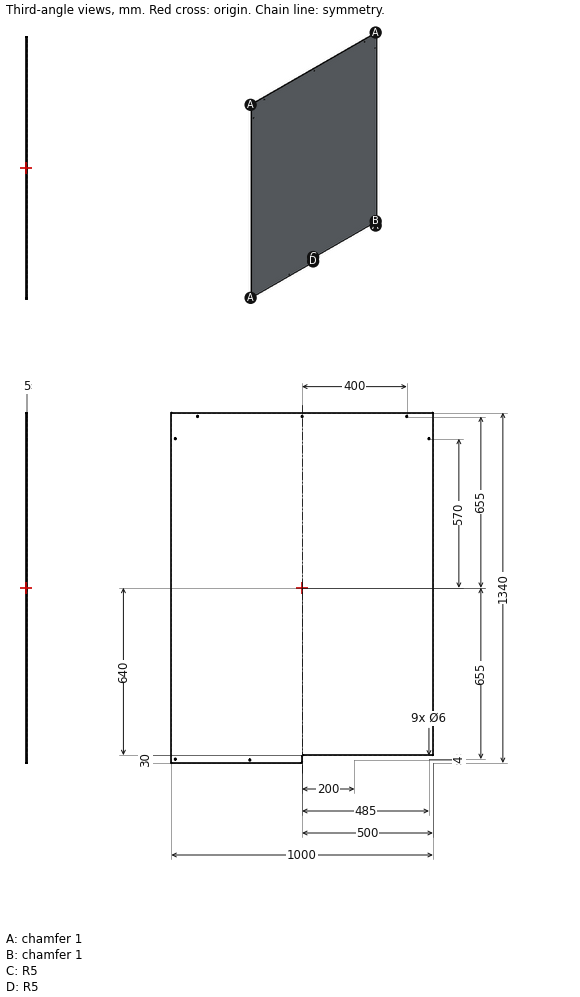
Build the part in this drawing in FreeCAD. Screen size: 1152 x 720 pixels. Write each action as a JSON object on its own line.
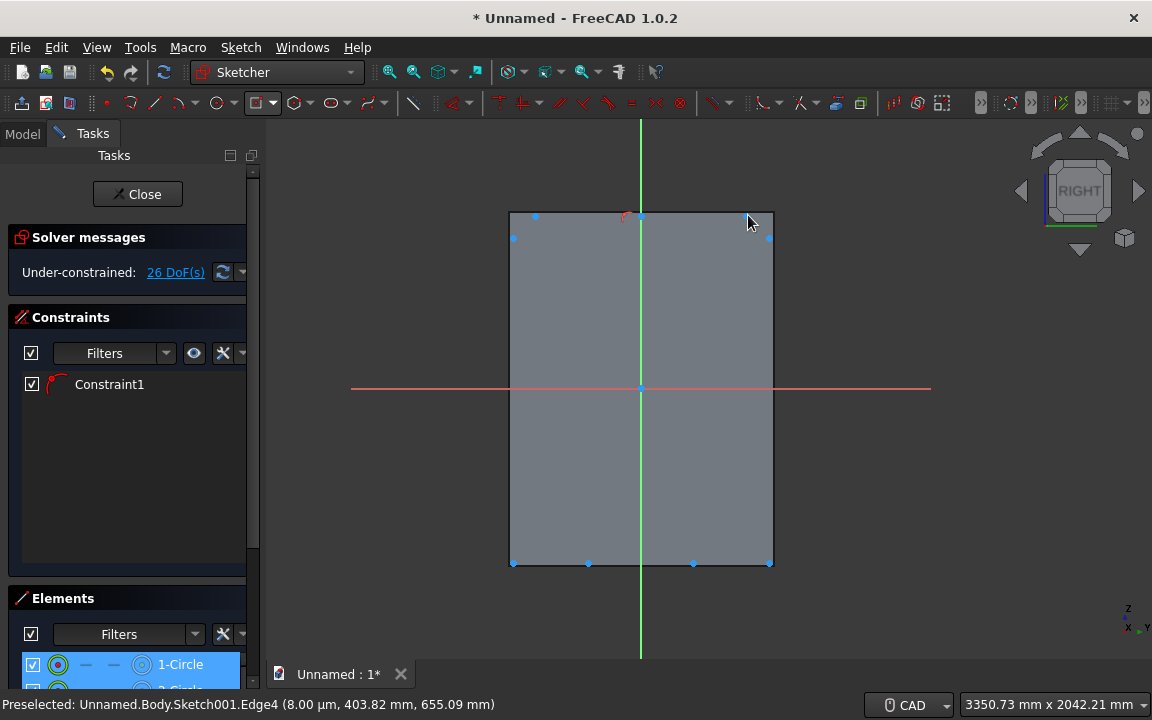
{"action": "scroll", "coordinate": [537, 216], "scroll_direction": "up", "scroll_amount": 10}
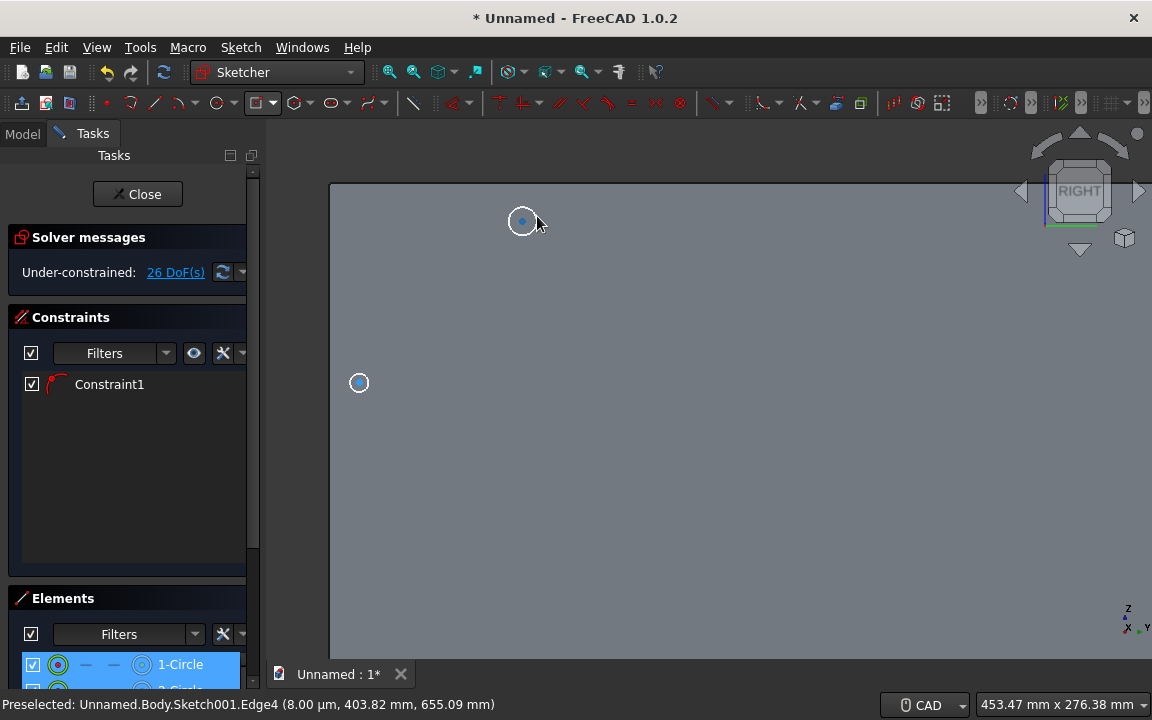
{"action": "left_click", "coordinate": [533, 211]}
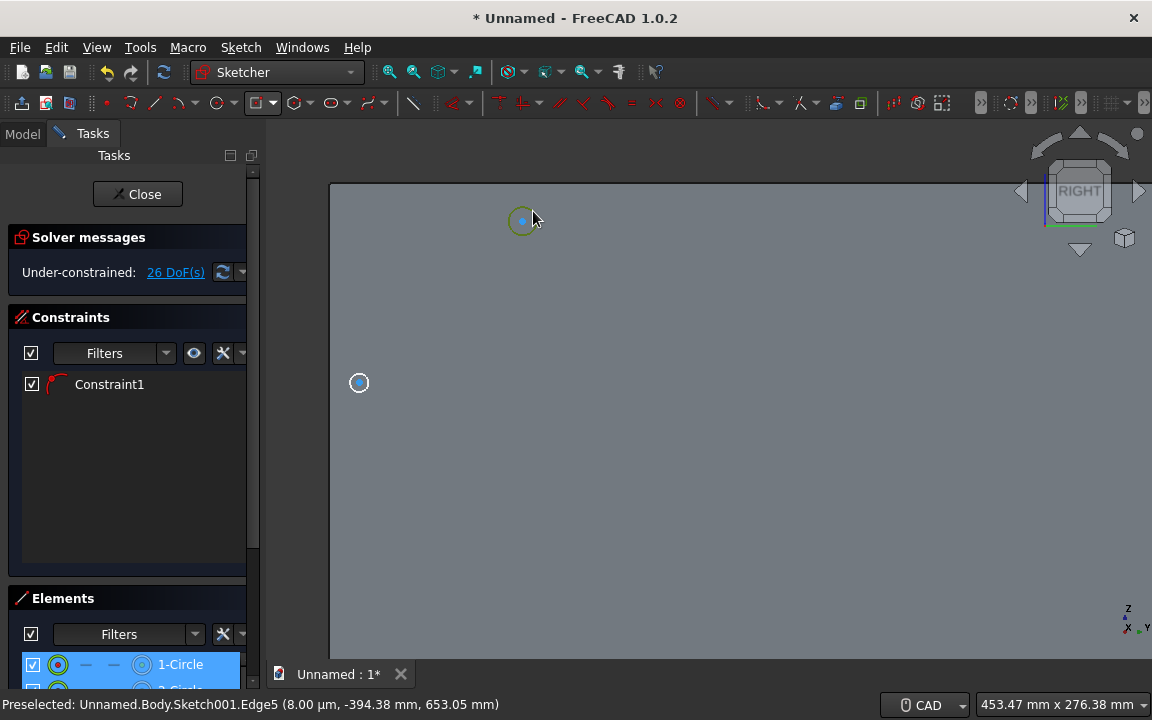
{"action": "scroll", "coordinate": [366, 376], "scroll_direction": "up", "scroll_amount": 3}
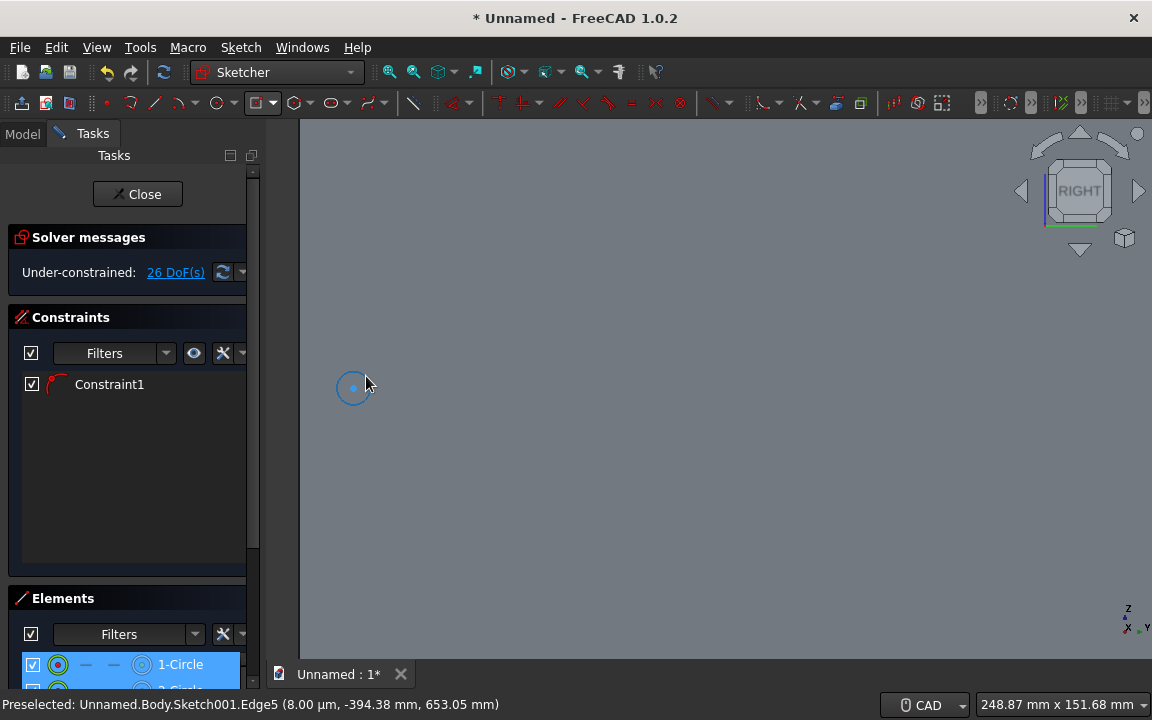
{"action": "left_click", "coordinate": [365, 376]}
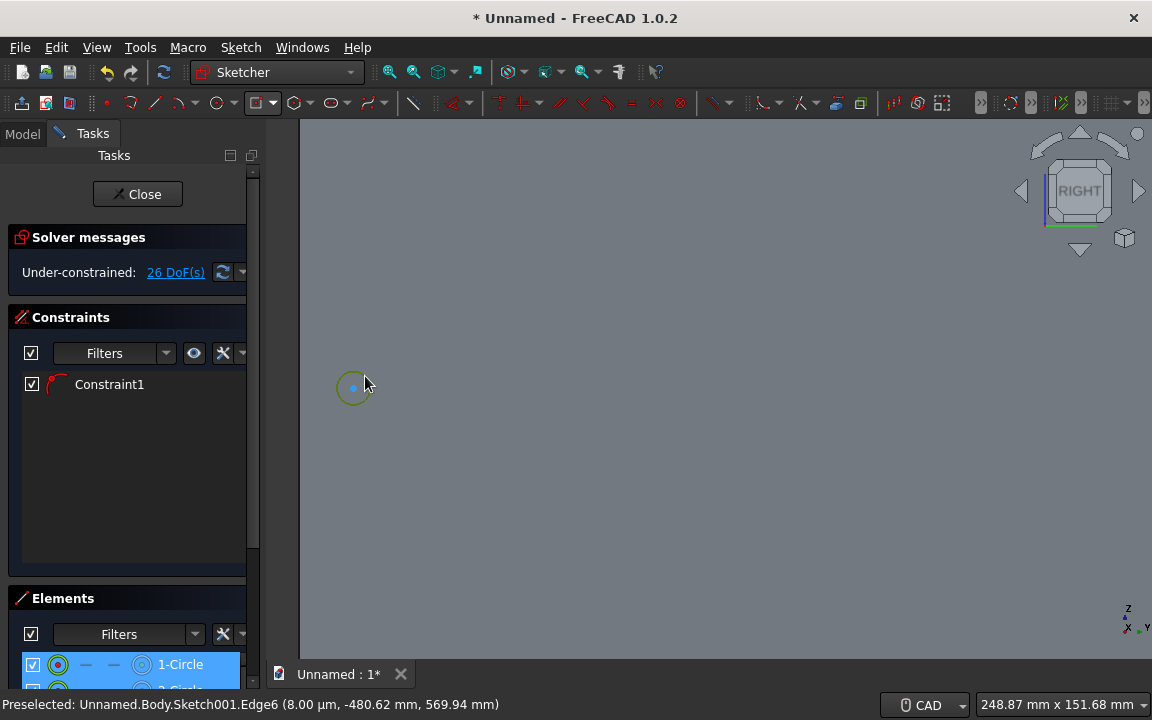
{"action": "scroll", "coordinate": [525, 226], "scroll_direction": "down", "scroll_amount": 13}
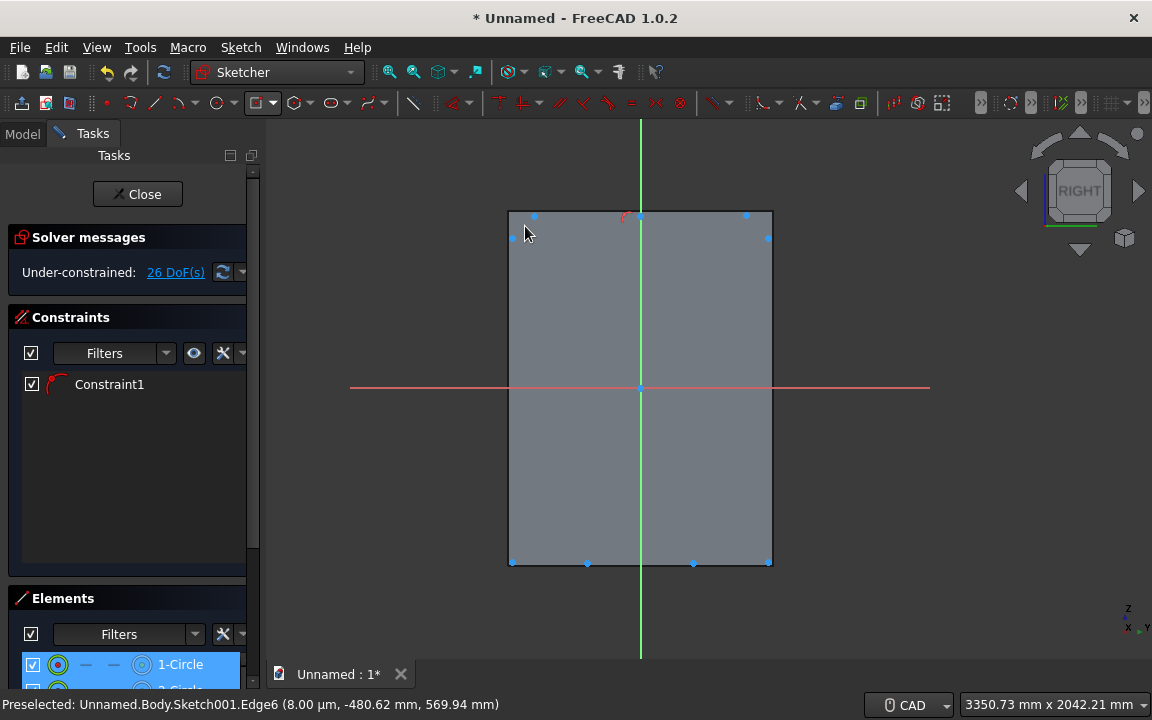
{"action": "scroll", "coordinate": [642, 215], "scroll_direction": "up", "scroll_amount": 13}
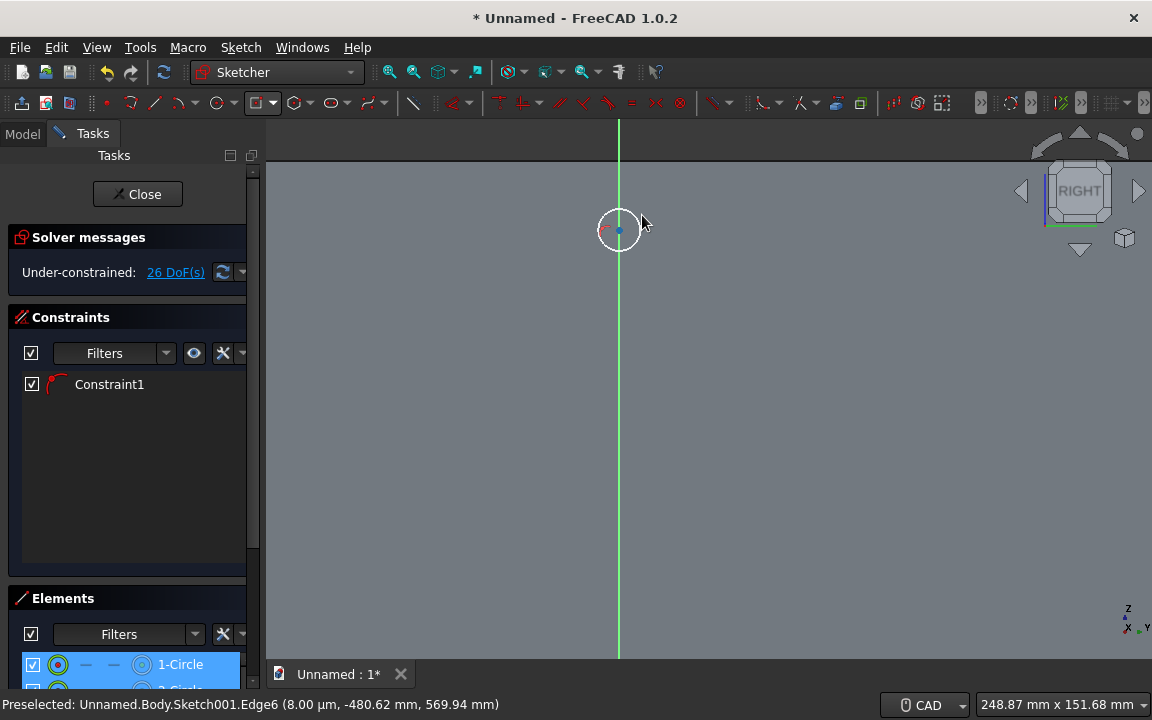
{"action": "left_click", "coordinate": [634, 215]}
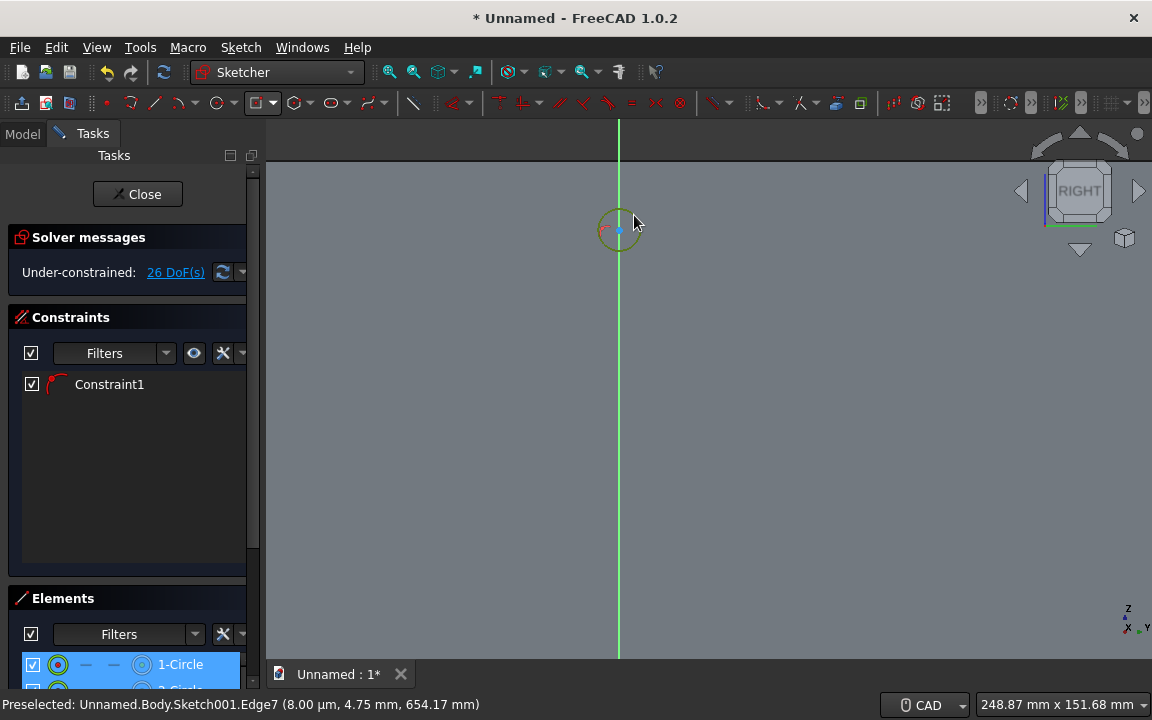
{"action": "scroll", "coordinate": [642, 215], "scroll_direction": "down", "scroll_amount": 13}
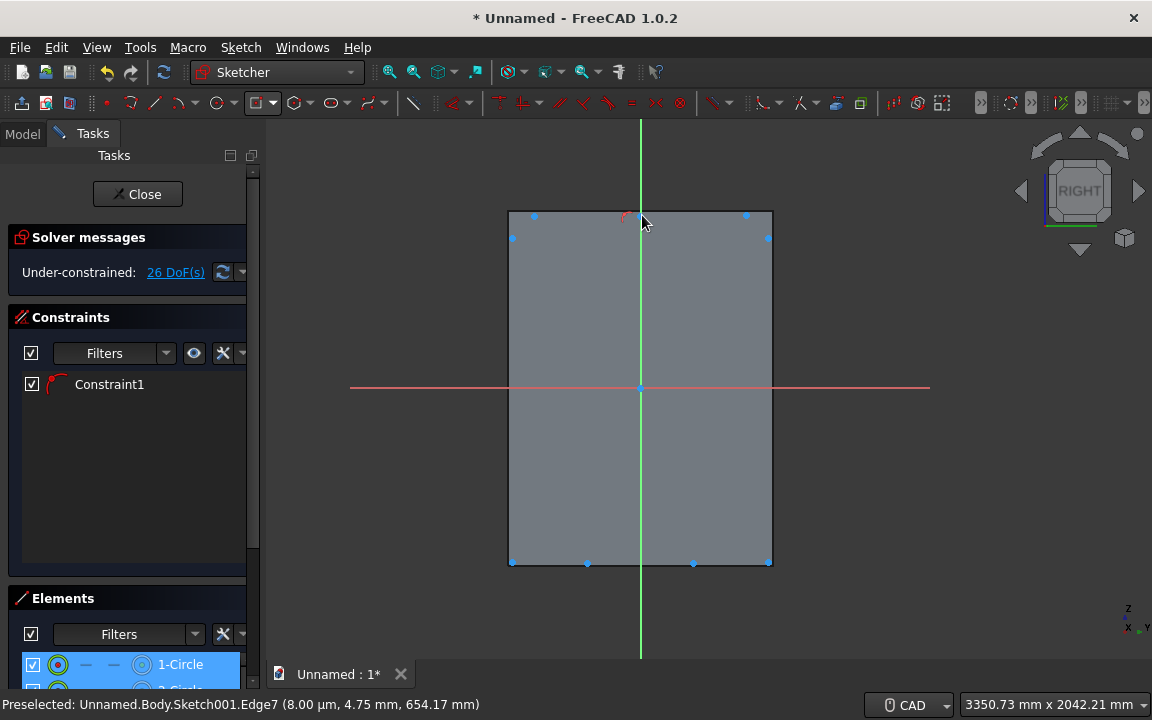
{"action": "scroll", "coordinate": [694, 562], "scroll_direction": "up", "scroll_amount": 11}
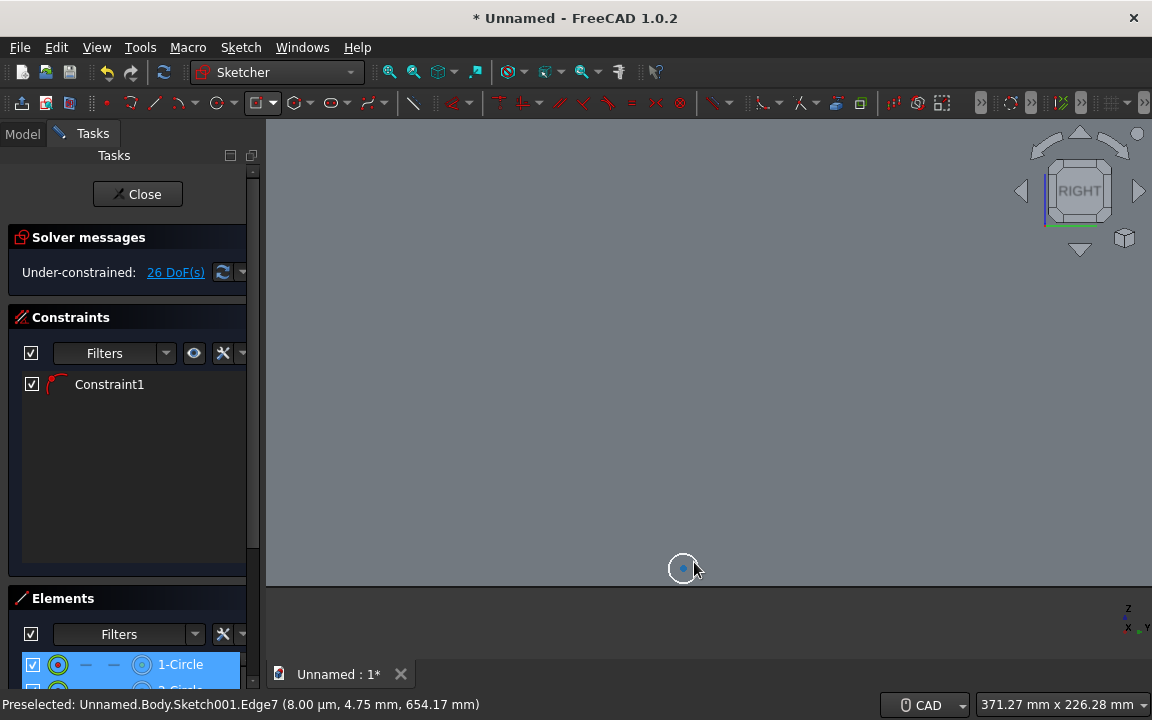
{"action": "left_click", "coordinate": [694, 558]}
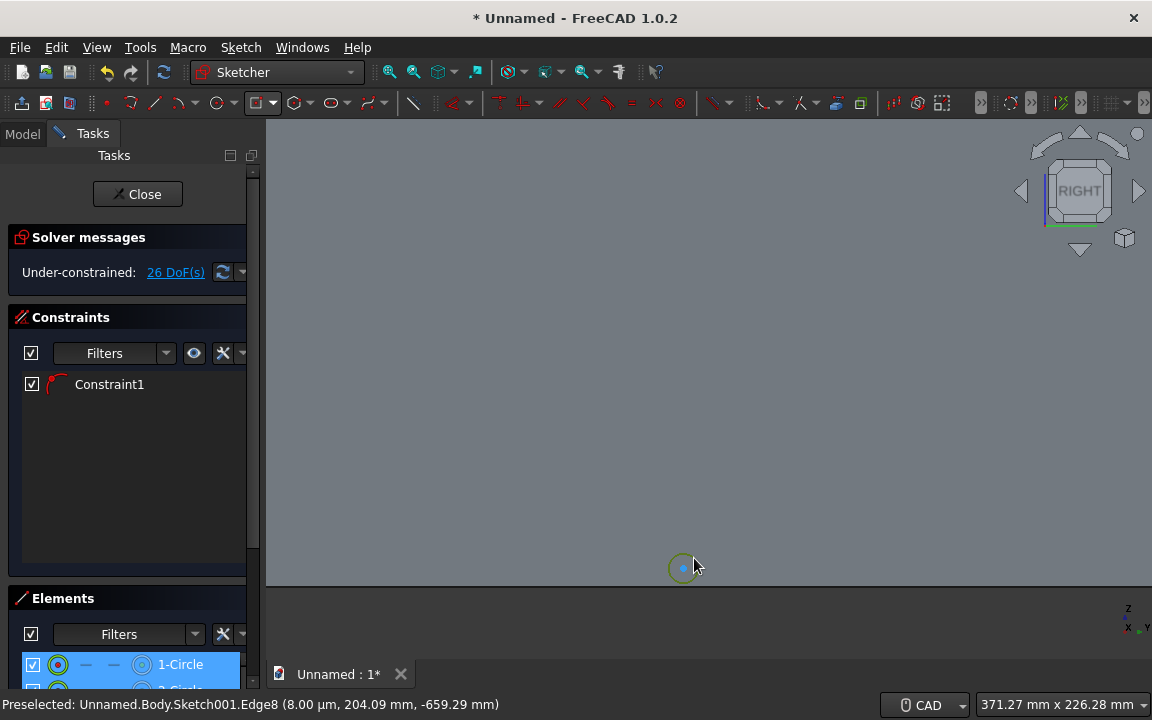
{"action": "scroll", "coordinate": [694, 563], "scroll_direction": "down", "scroll_amount": 11}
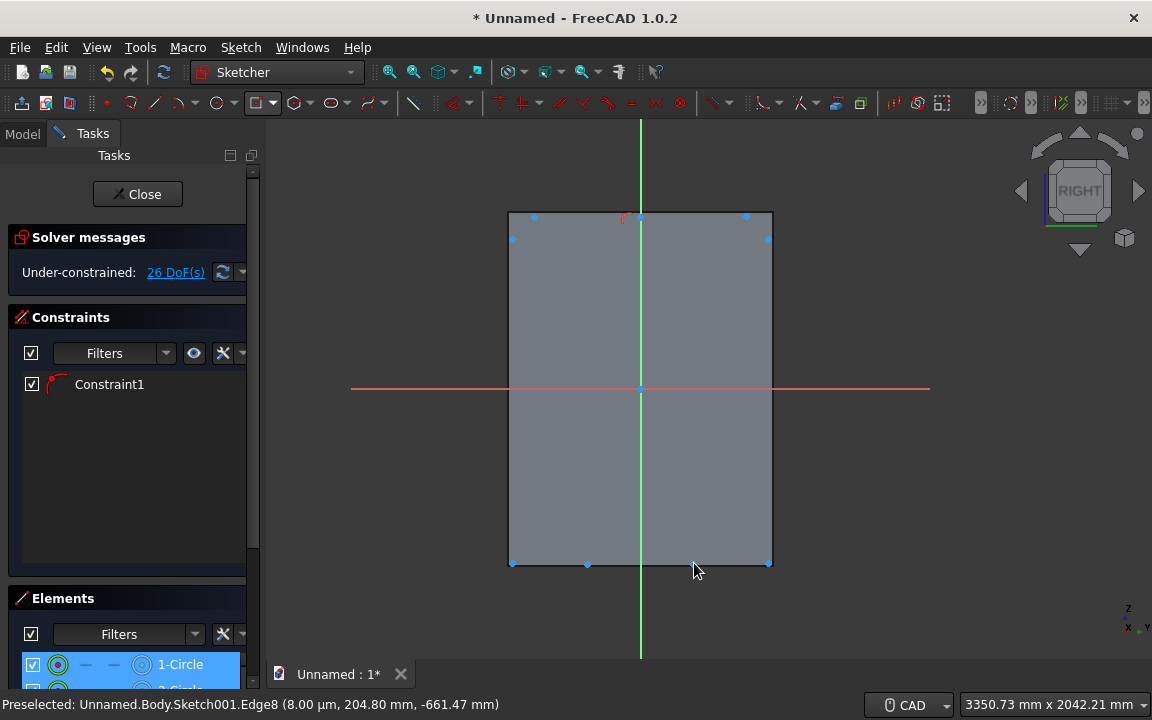
{"action": "scroll", "coordinate": [589, 563], "scroll_direction": "up", "scroll_amount": 12}